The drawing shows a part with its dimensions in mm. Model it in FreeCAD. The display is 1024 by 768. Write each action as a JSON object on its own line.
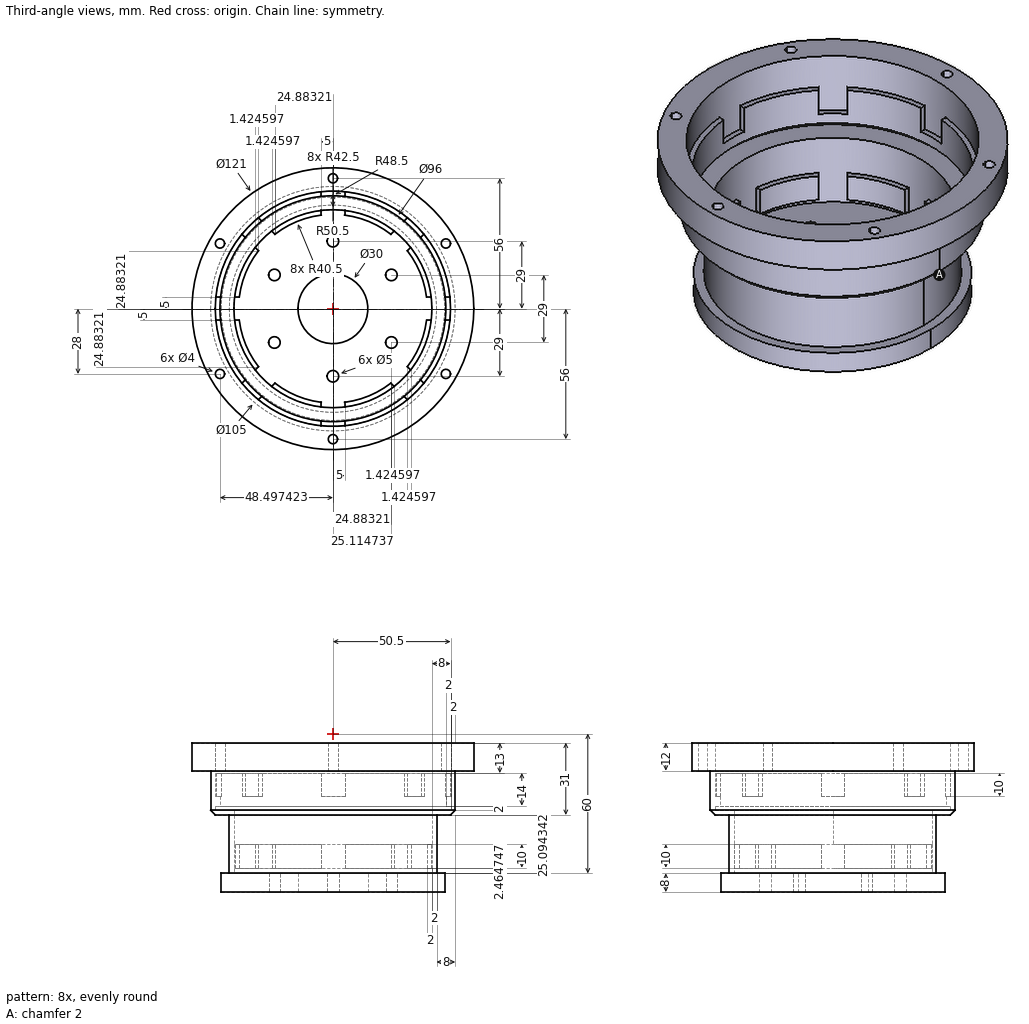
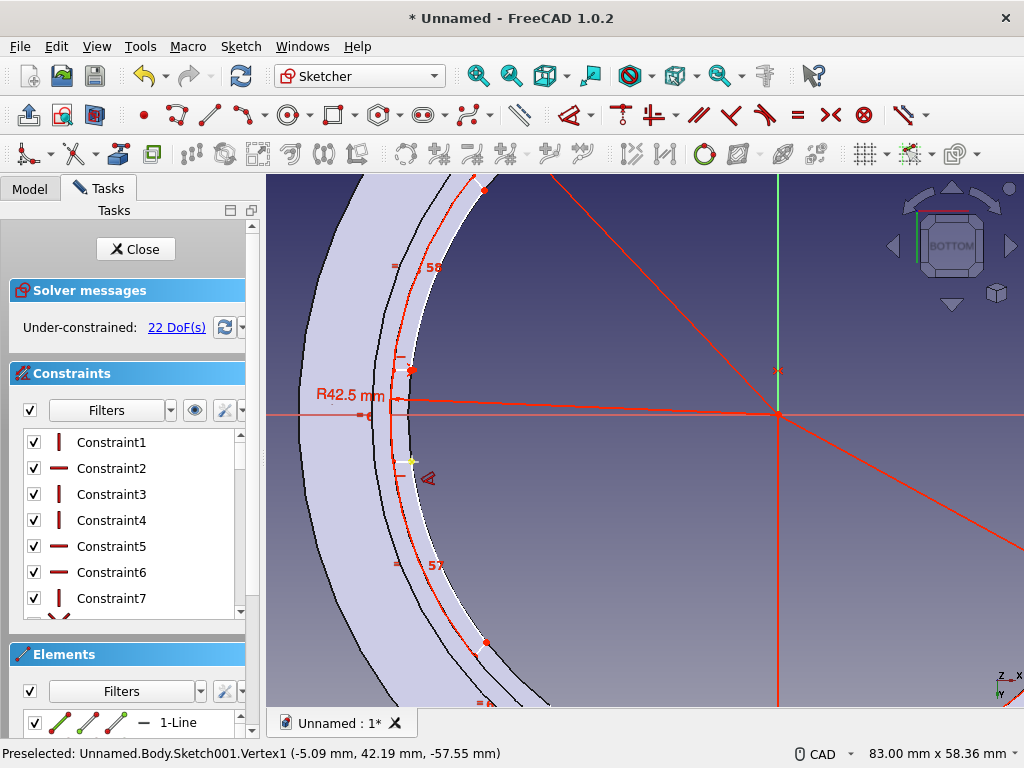
{"action": "left_click", "coordinate": [411, 462]}
{"action": "left_click", "coordinate": [377, 438]}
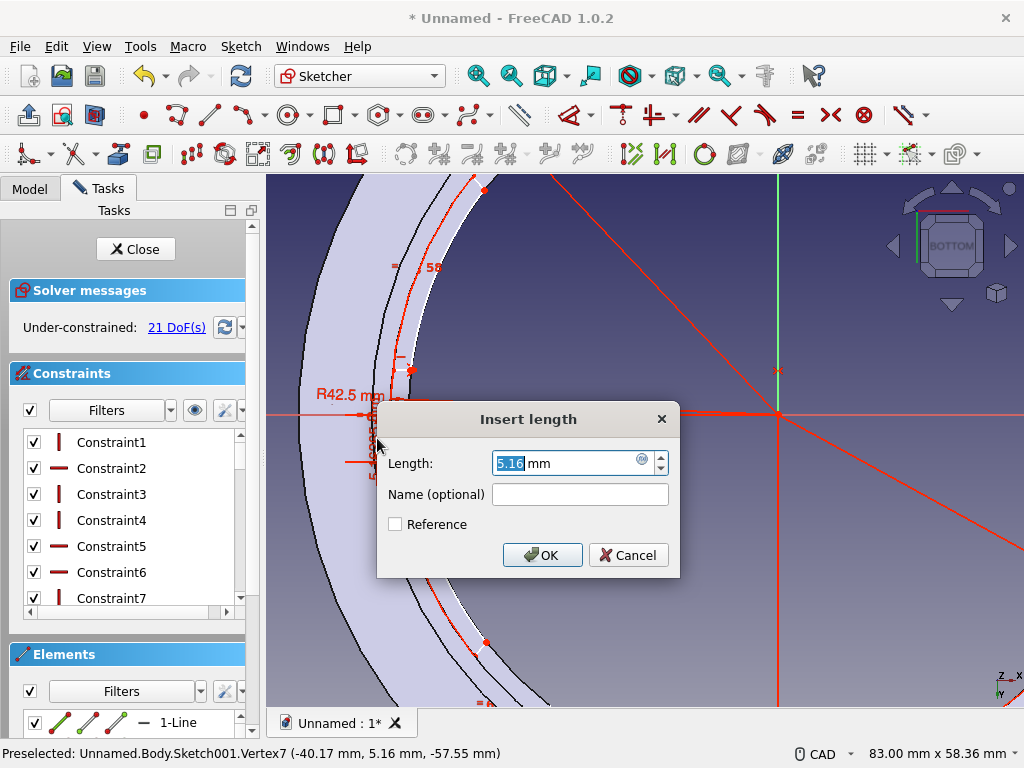
{"action": "type", "text": "5"}
{"action": "key", "text": "Return"}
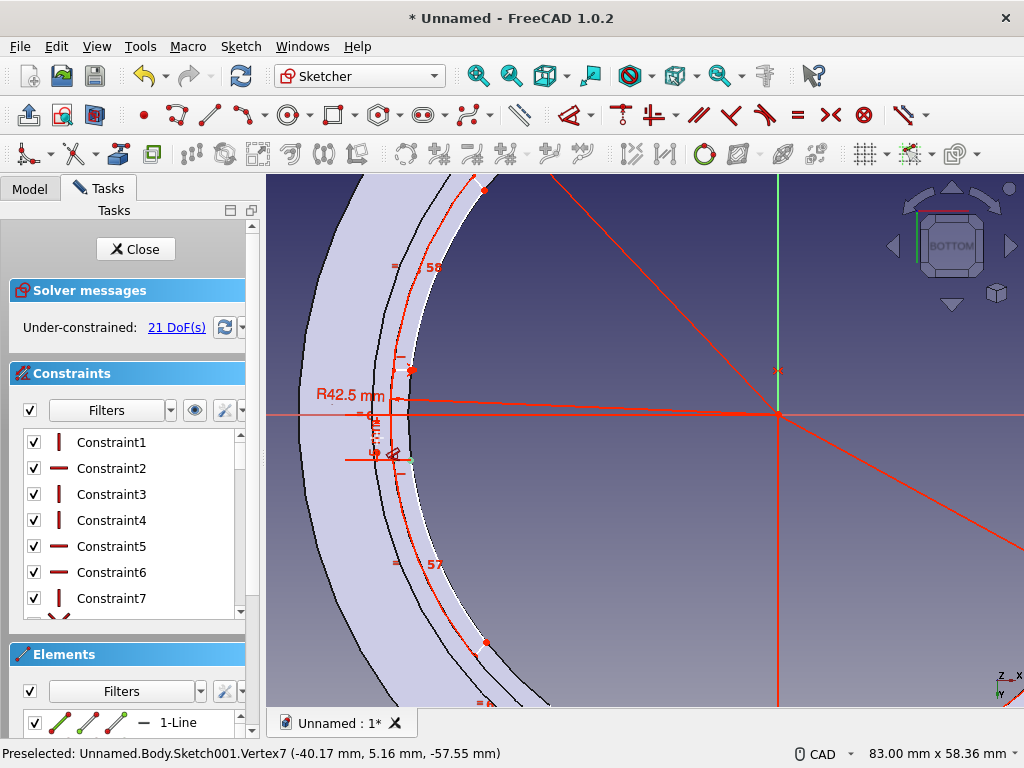
{"action": "left_click", "coordinate": [392, 370]}
{"action": "left_click", "coordinate": [812, 392]}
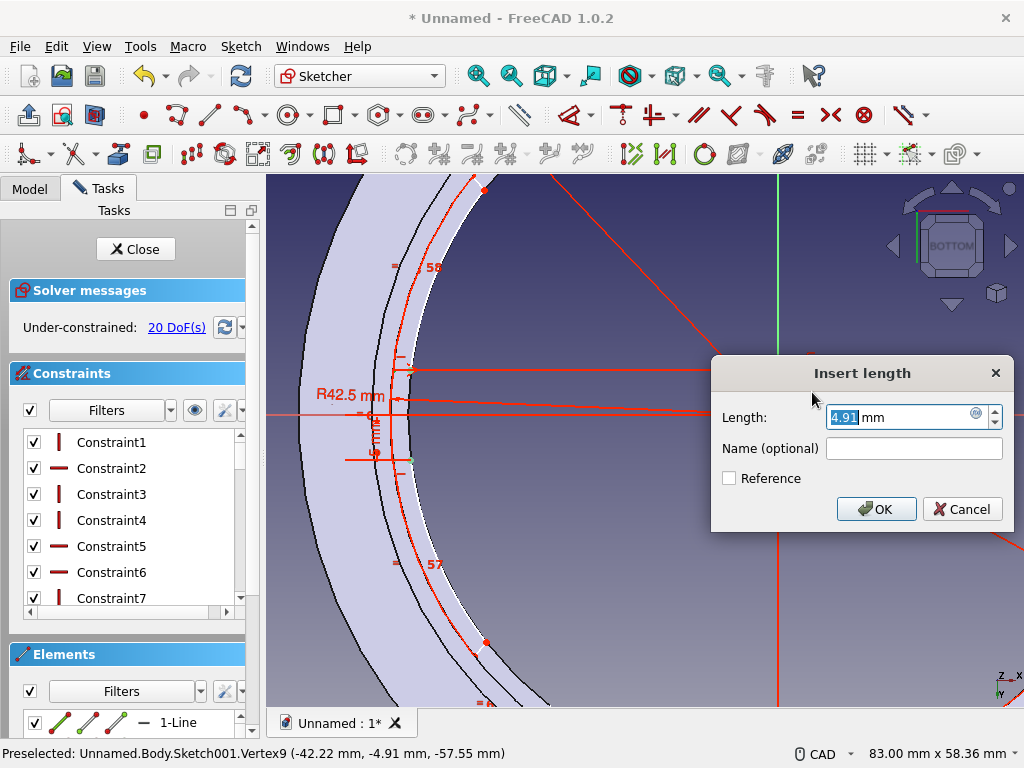
{"action": "type", "text": "5"}
{"action": "key", "text": "Return"}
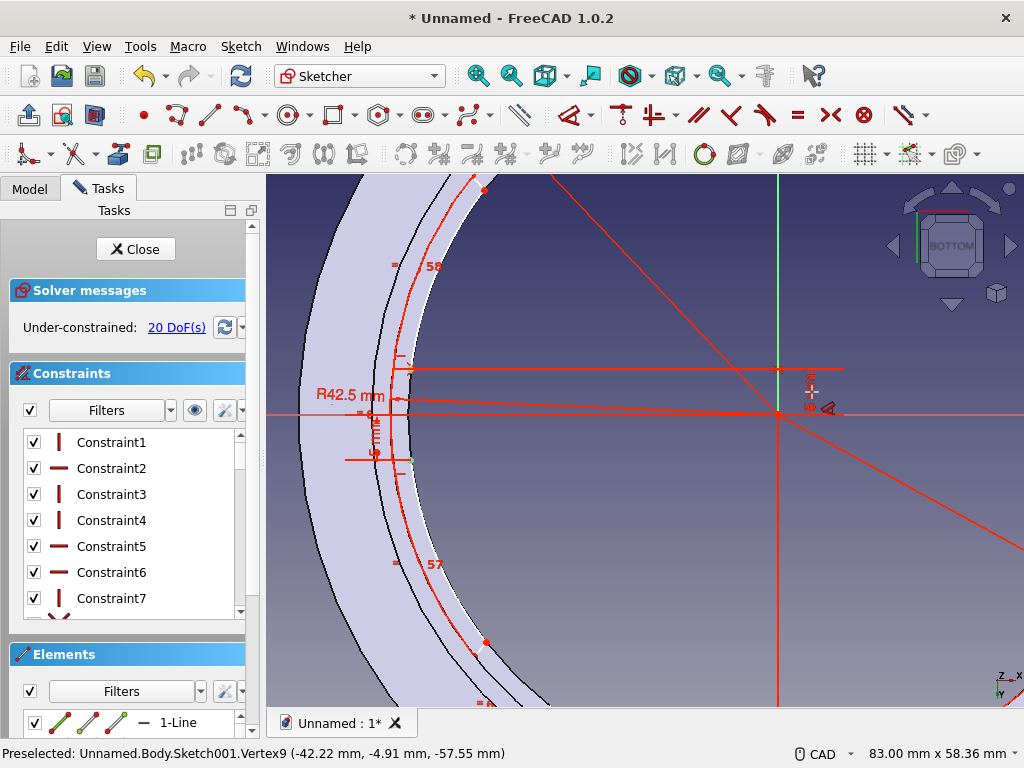
{"action": "scroll", "coordinate": [412, 461], "scroll_direction": "down", "scroll_amount": 4}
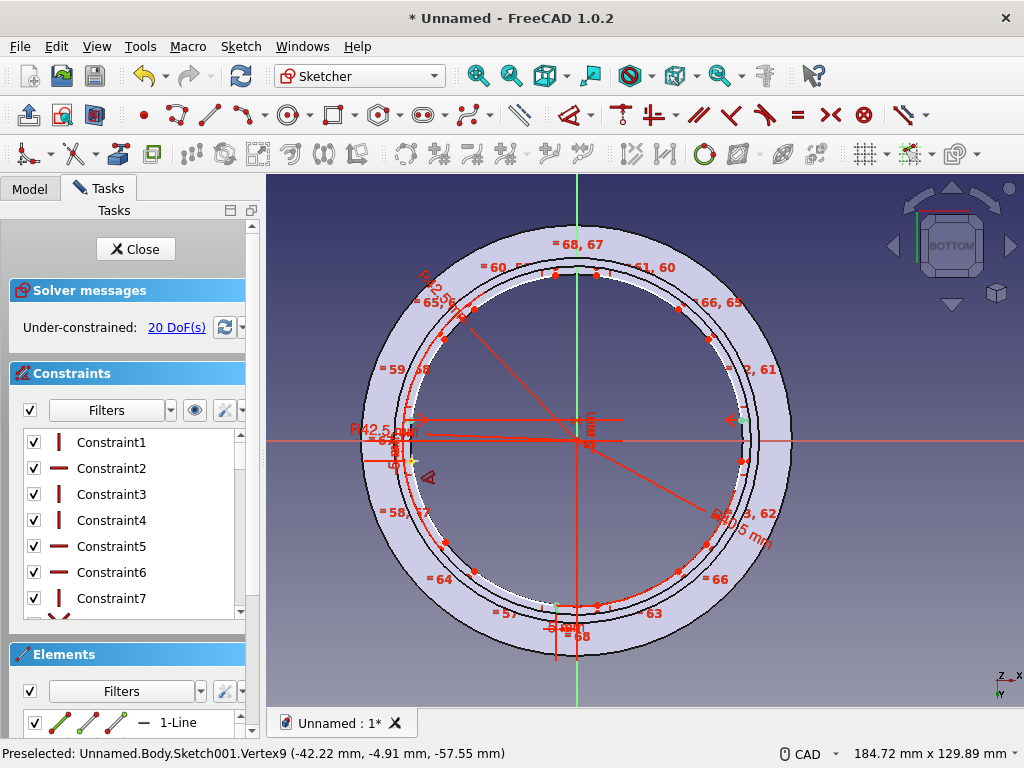
{"action": "scroll", "coordinate": [556, 276], "scroll_direction": "up", "scroll_amount": 4}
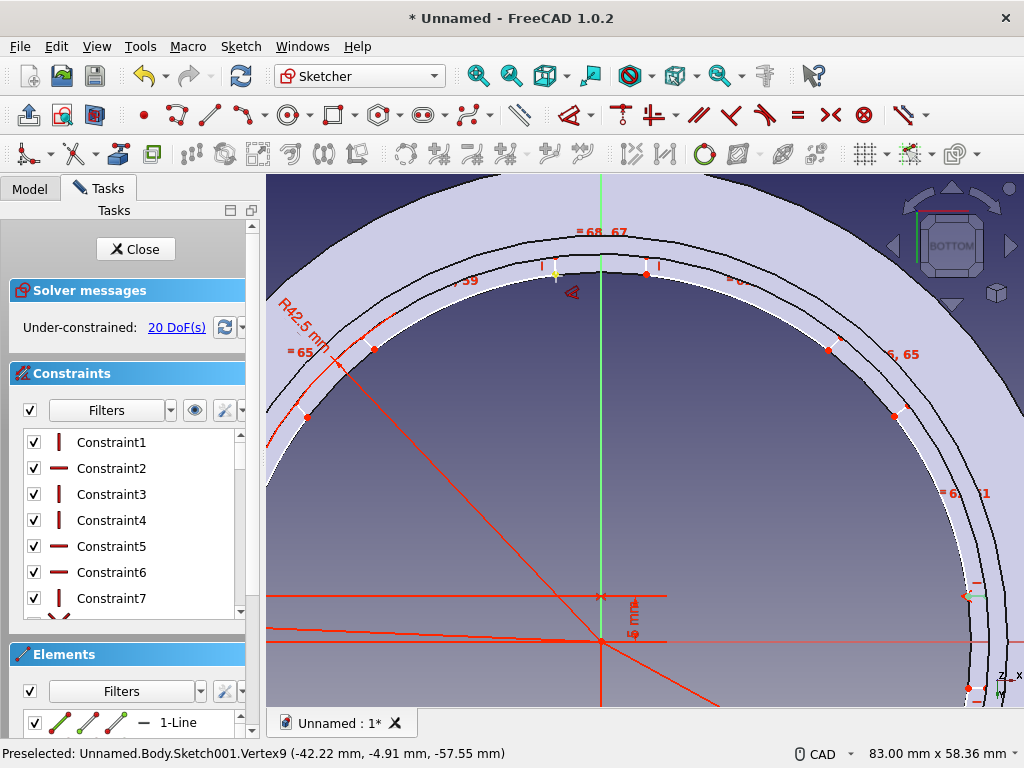
{"action": "left_click", "coordinate": [555, 275]}
{"action": "left_click", "coordinate": [578, 241]}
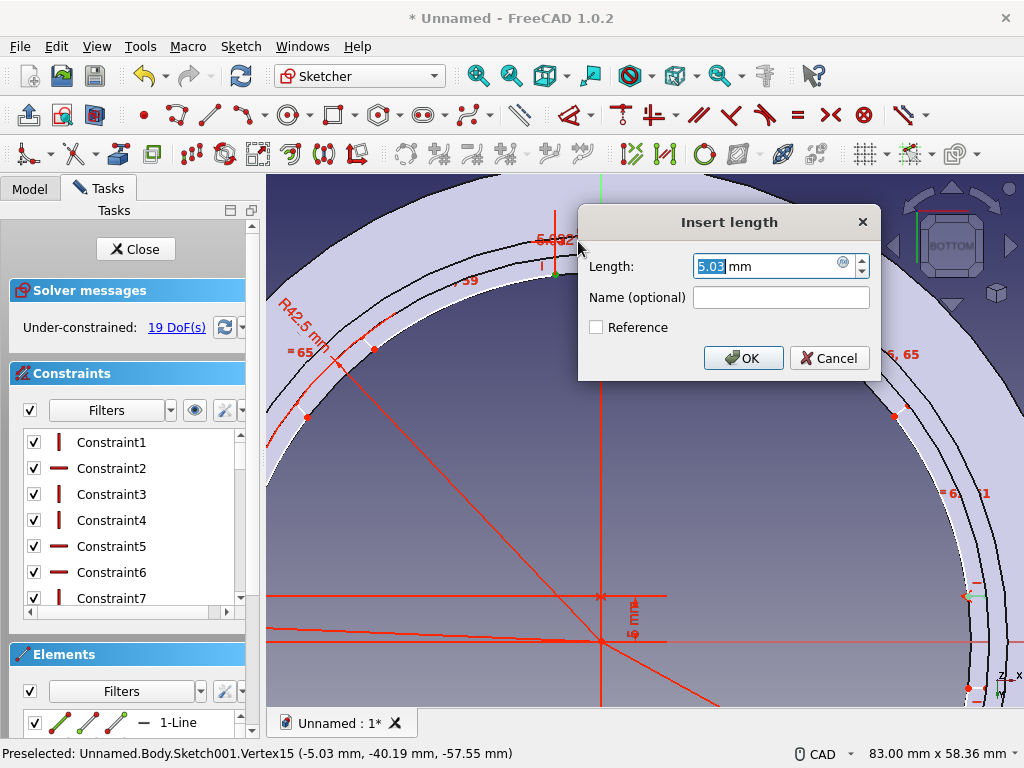
{"action": "type", "text": "5"}
{"action": "key", "text": "Return"}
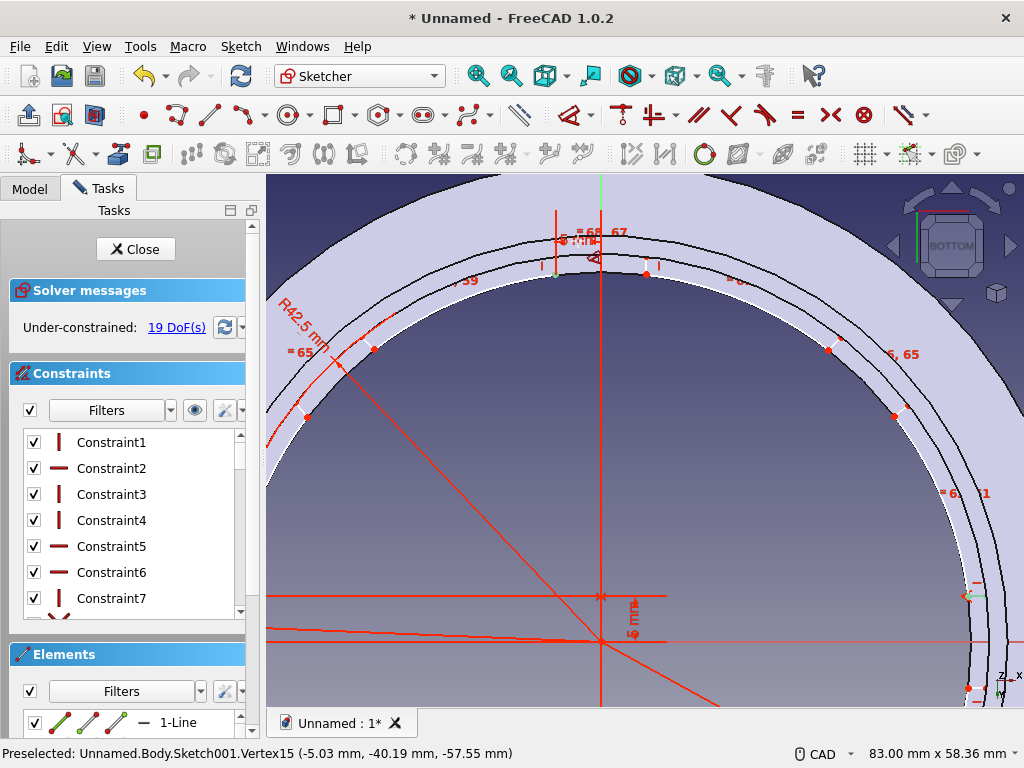
{"action": "left_click", "coordinate": [646, 256]}
{"action": "left_click", "coordinate": [624, 676]}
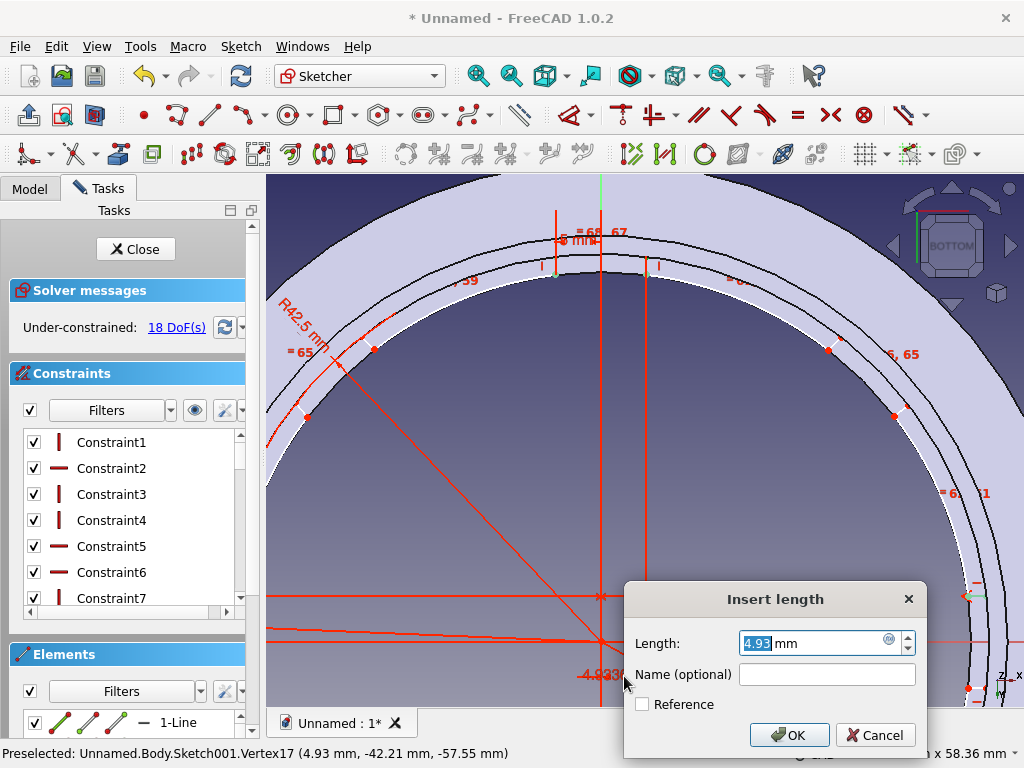
{"action": "type", "text": "5"}
{"action": "key", "text": "Return"}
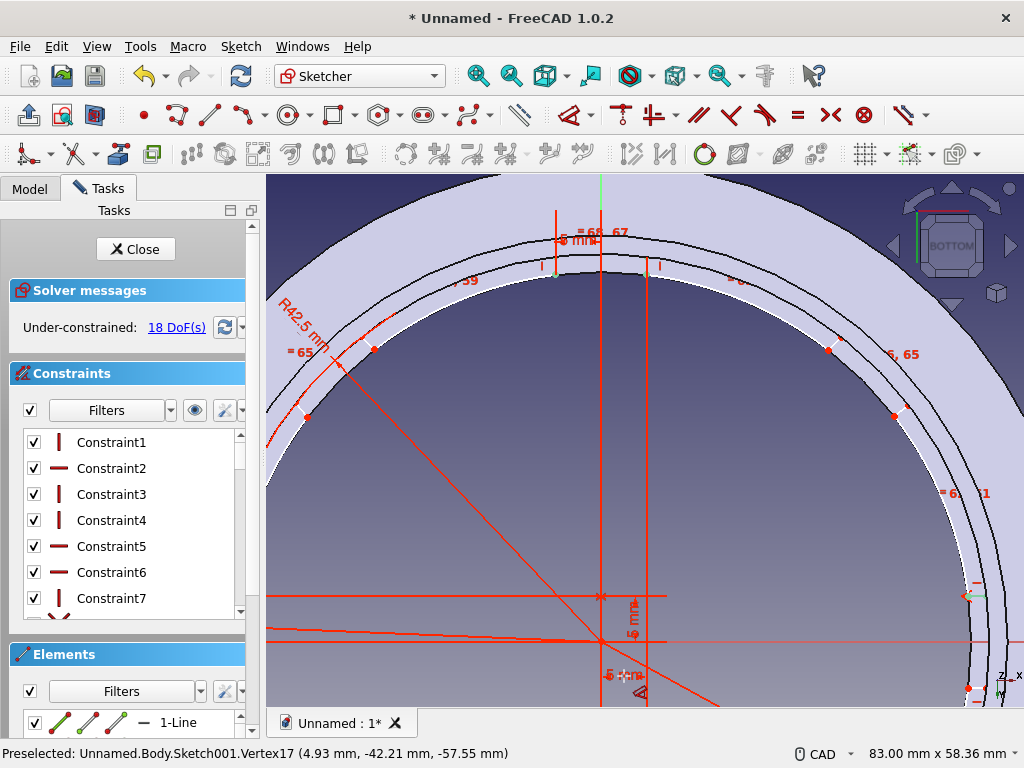
{"action": "scroll", "coordinate": [556, 276], "scroll_direction": "down", "scroll_amount": 4}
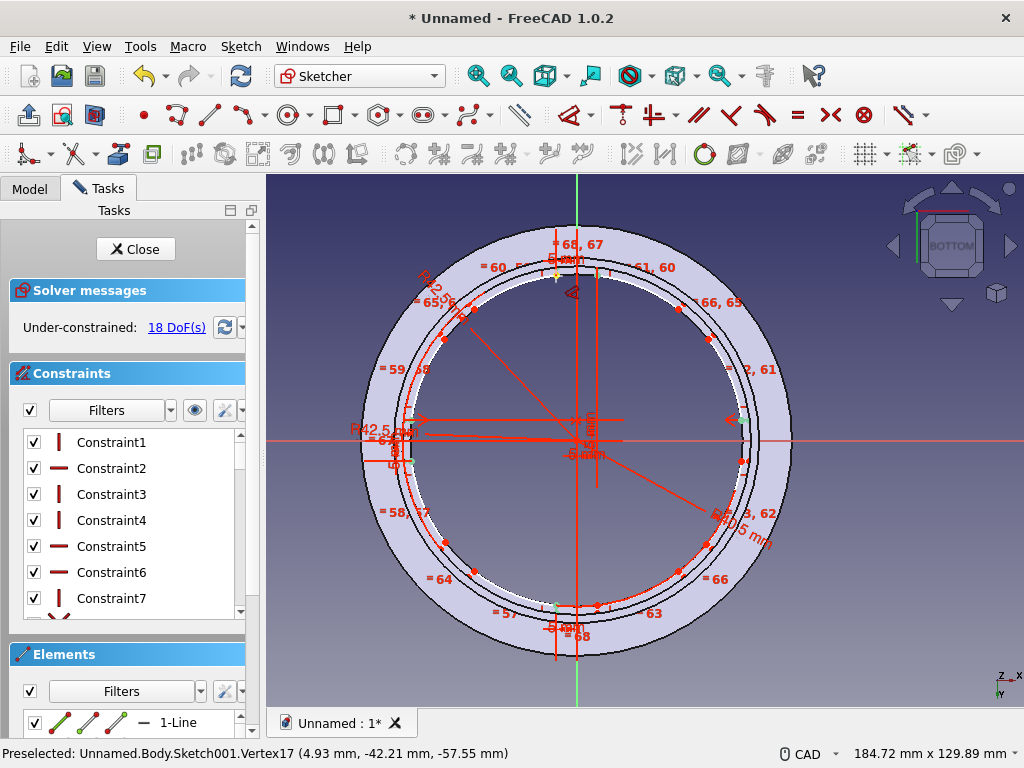
{"action": "scroll", "coordinate": [750, 461], "scroll_direction": "up", "scroll_amount": 4}